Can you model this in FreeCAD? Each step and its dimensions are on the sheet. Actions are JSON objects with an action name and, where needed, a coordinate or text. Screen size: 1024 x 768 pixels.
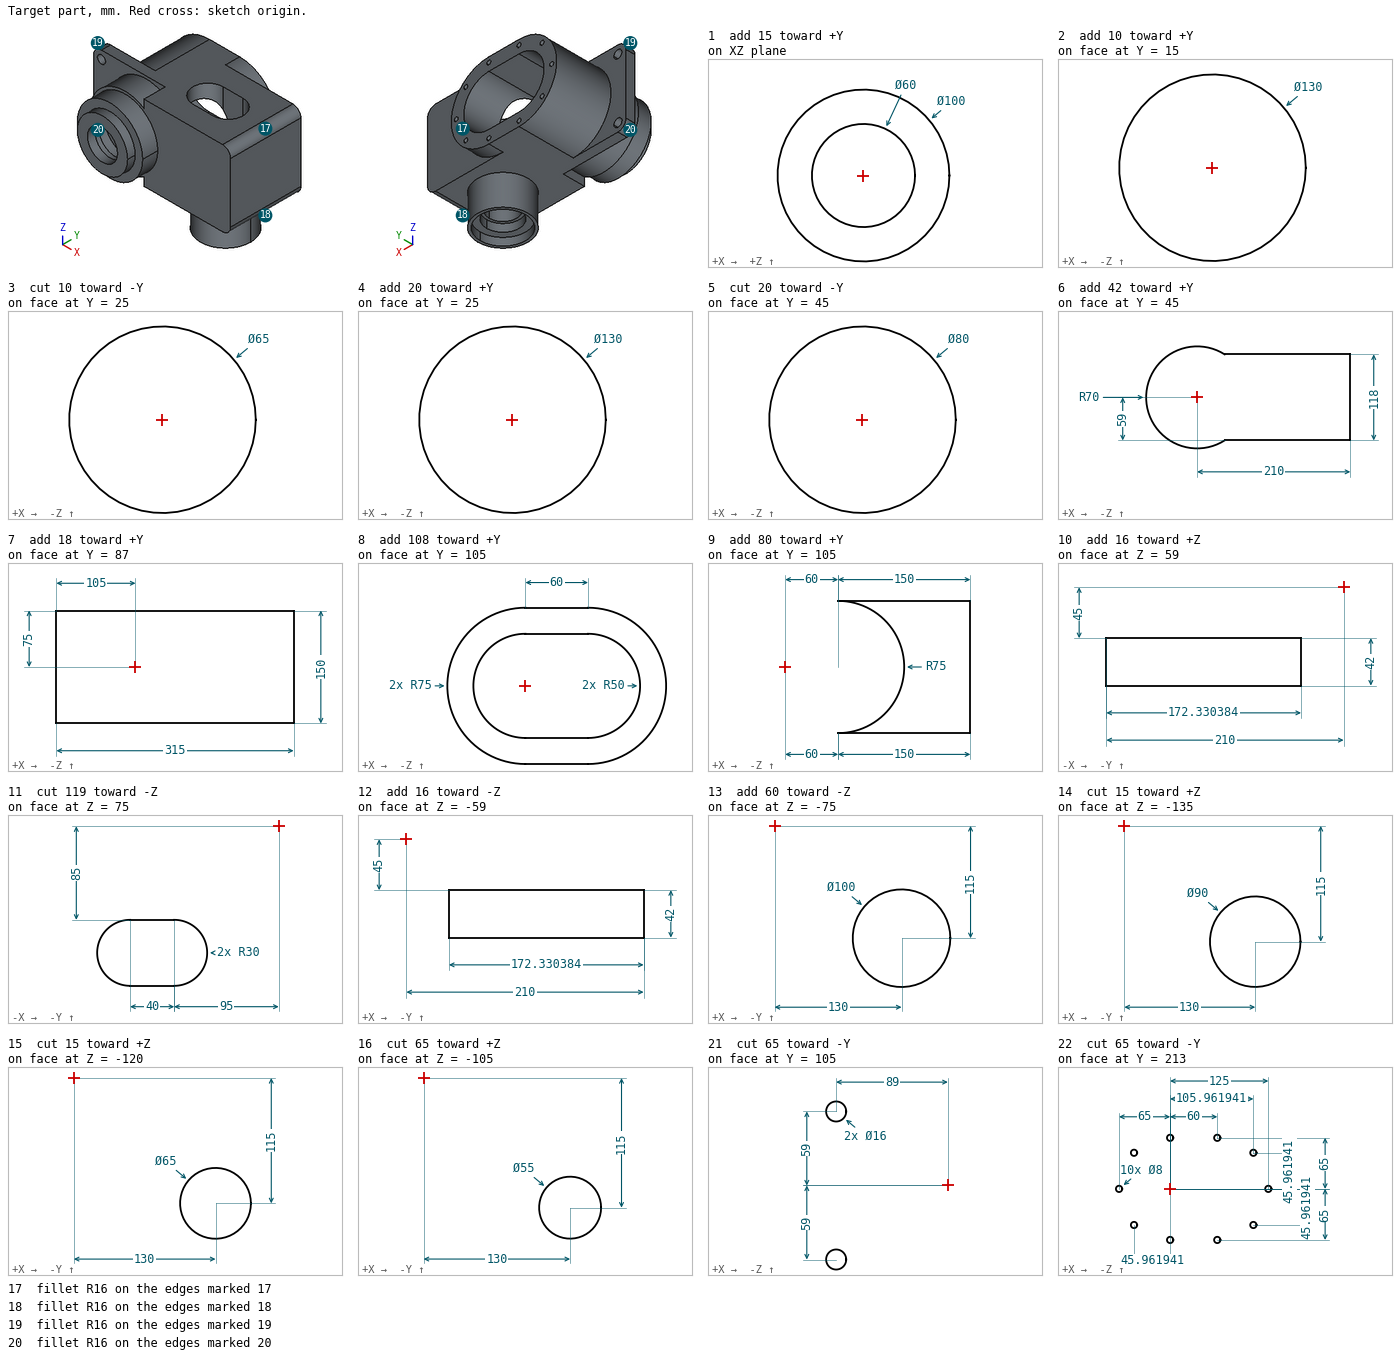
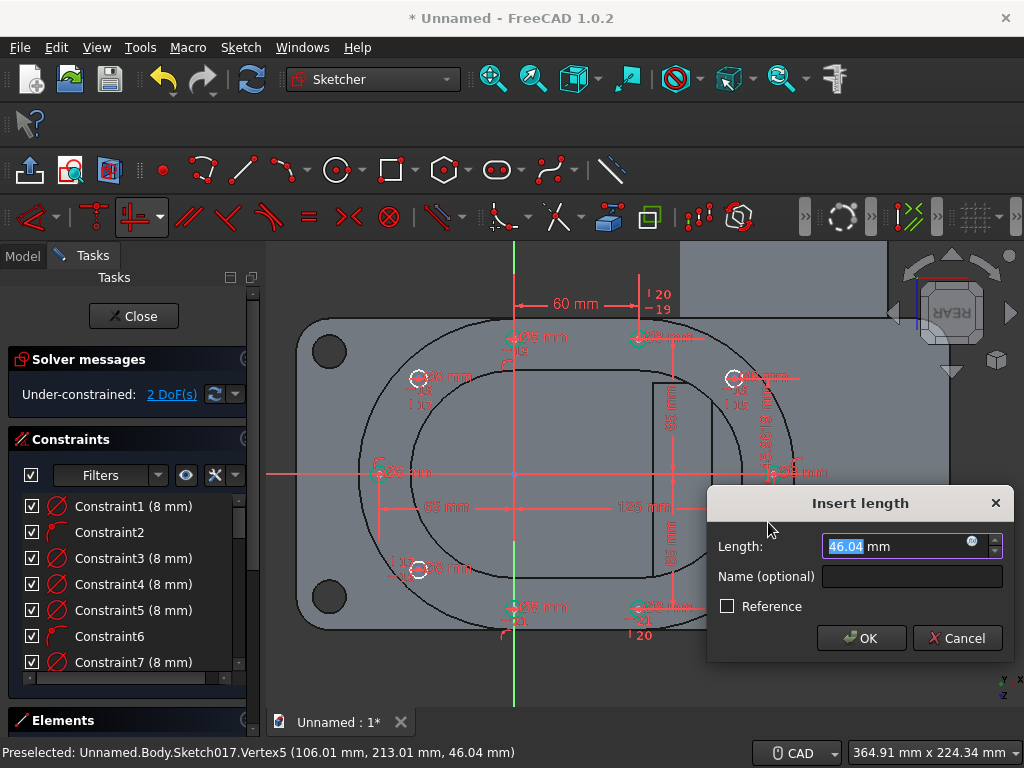
{"action": "type", "text": "45.961941"}
{"action": "key", "text": "Return"}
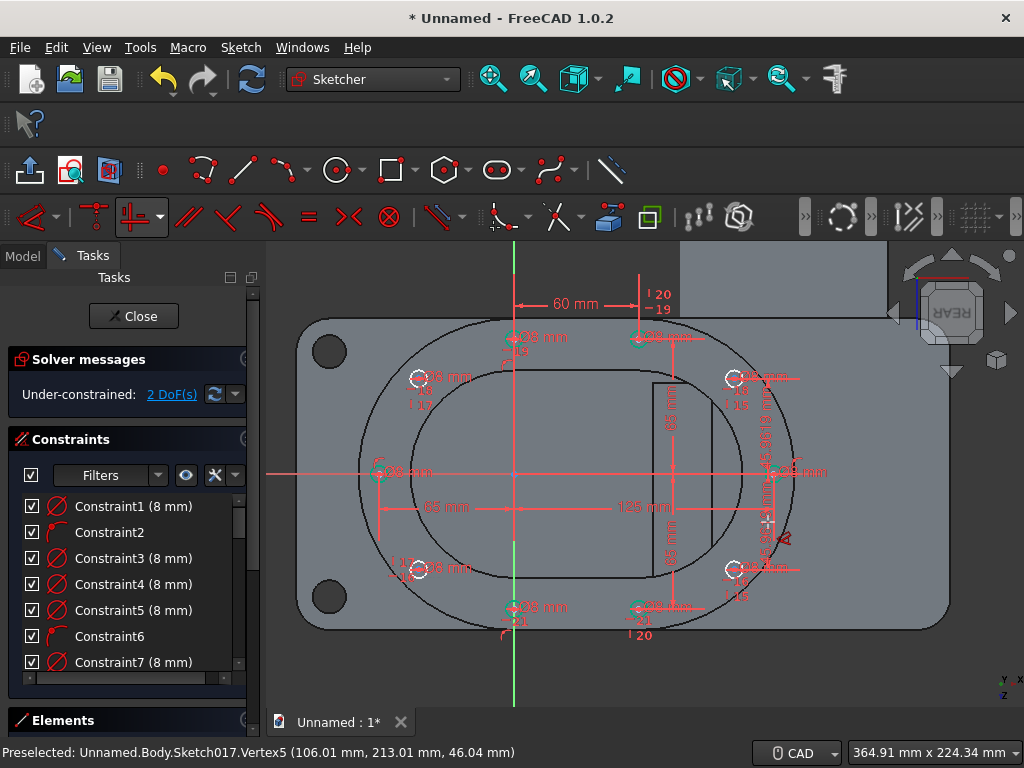
{"action": "left_click", "coordinate": [419, 570]}
{"action": "left_click", "coordinate": [466, 604]}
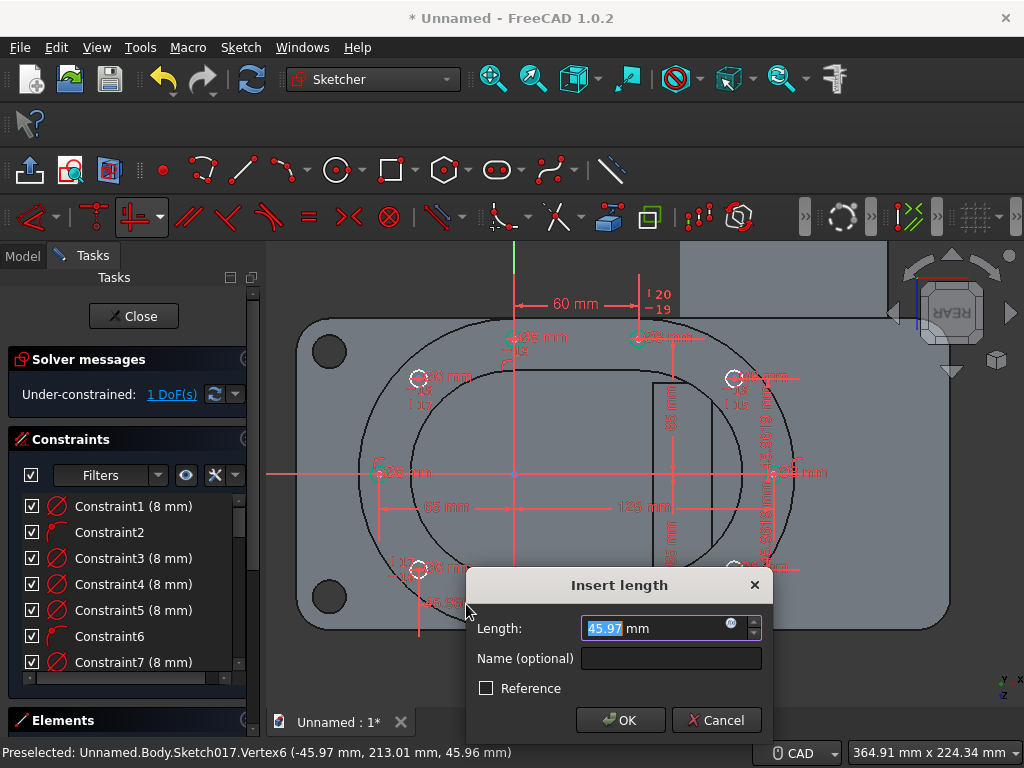
{"action": "type", "text": "45.961941"}
{"action": "key", "text": "Return"}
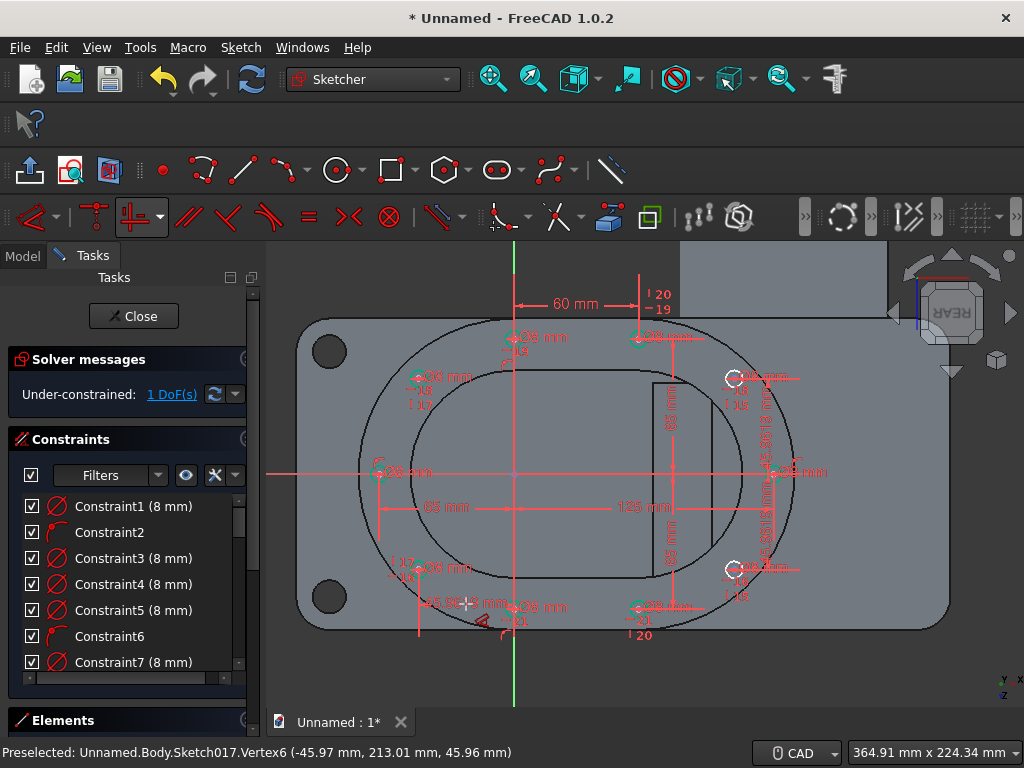
{"action": "left_click", "coordinate": [734, 379]}
{"action": "left_click", "coordinate": [574, 345]}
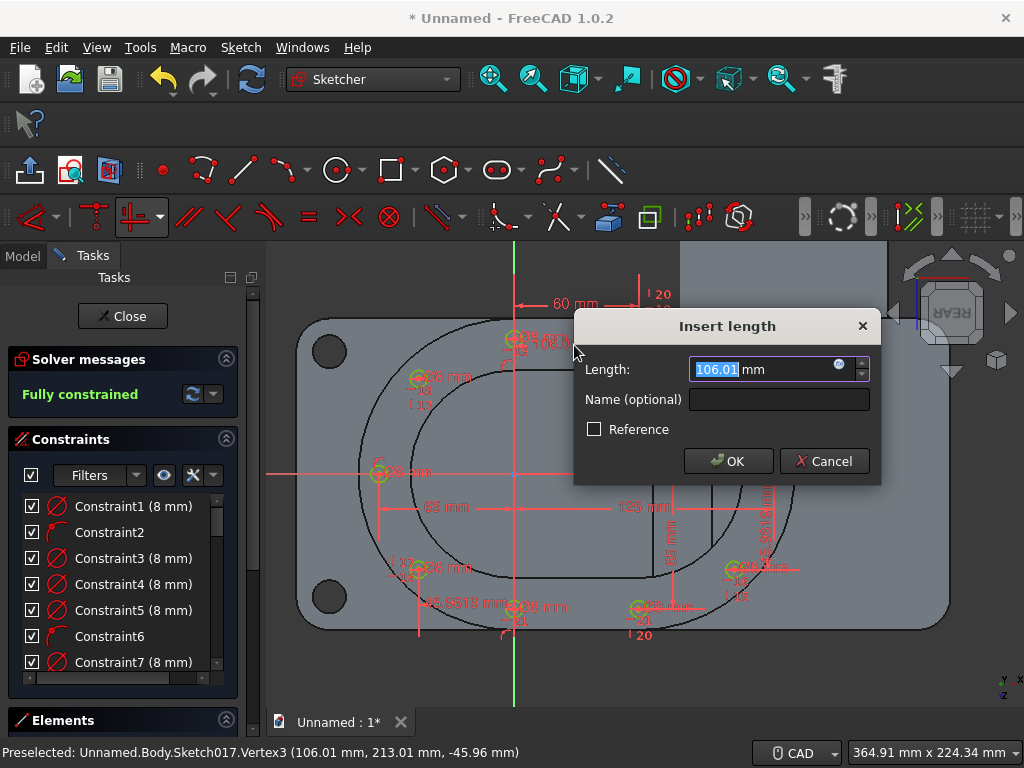
{"action": "type", "text": "105.961941"}
{"action": "key", "text": "Return"}
{"action": "key", "text": "Escape"}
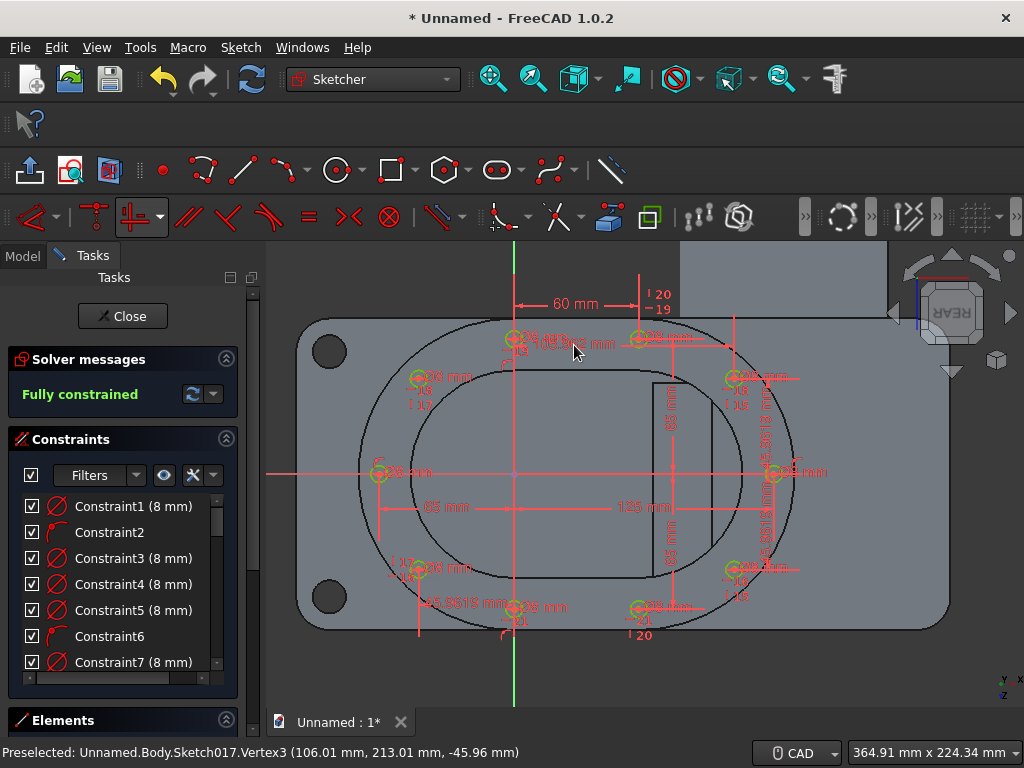
{"action": "left_click", "coordinate": [123, 316]}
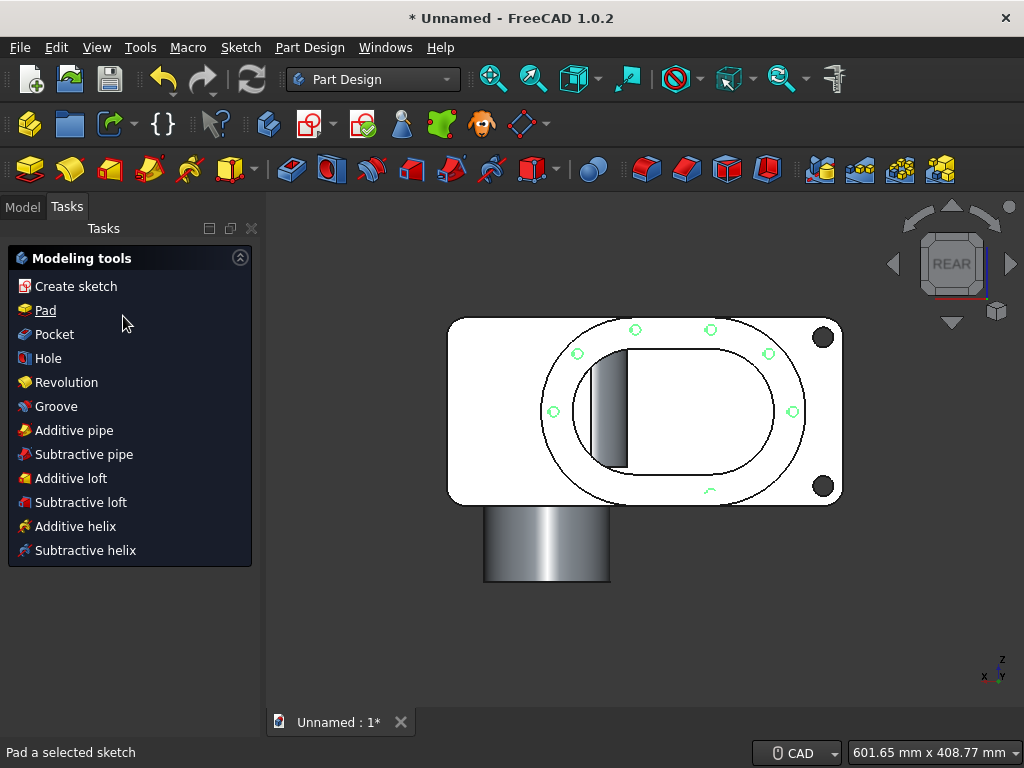
{"action": "left_click", "coordinate": [292, 170]}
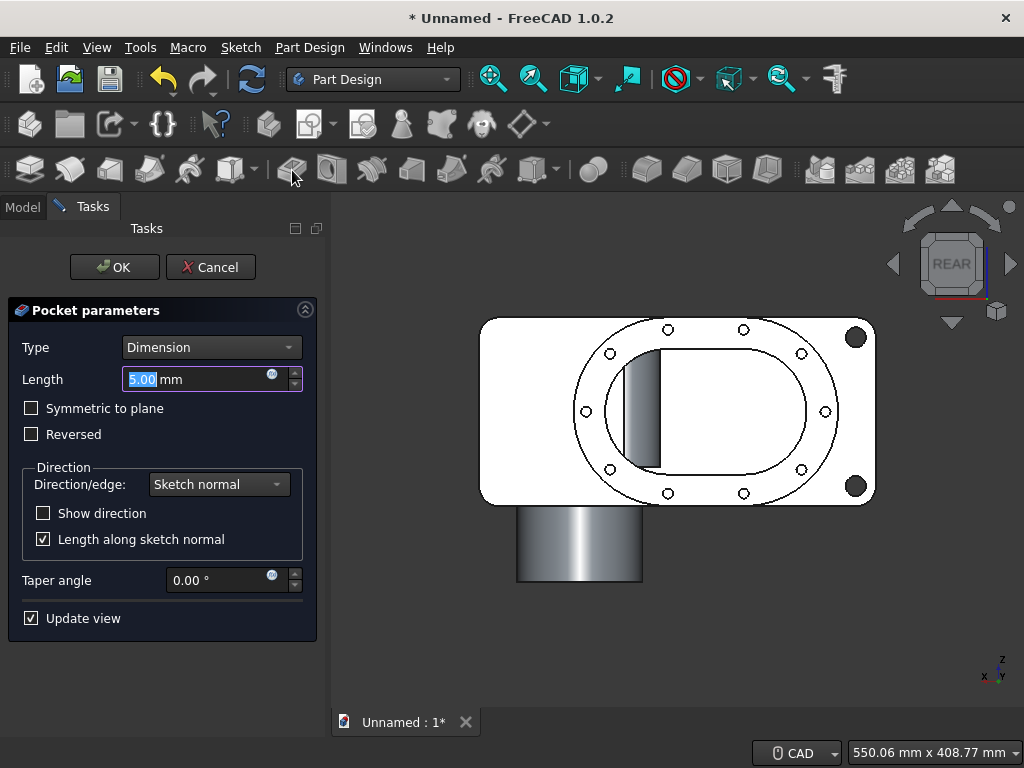
{"action": "type", "text": "65"}
{"action": "key", "text": "Tab"}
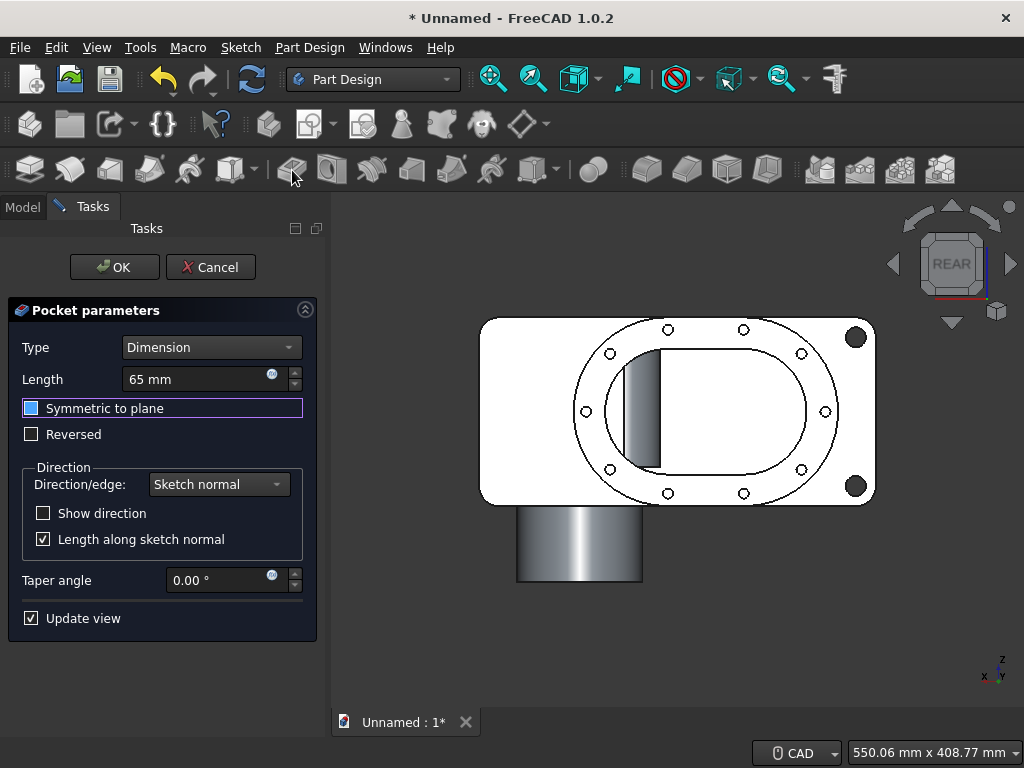
{"action": "left_click", "coordinate": [115, 267]}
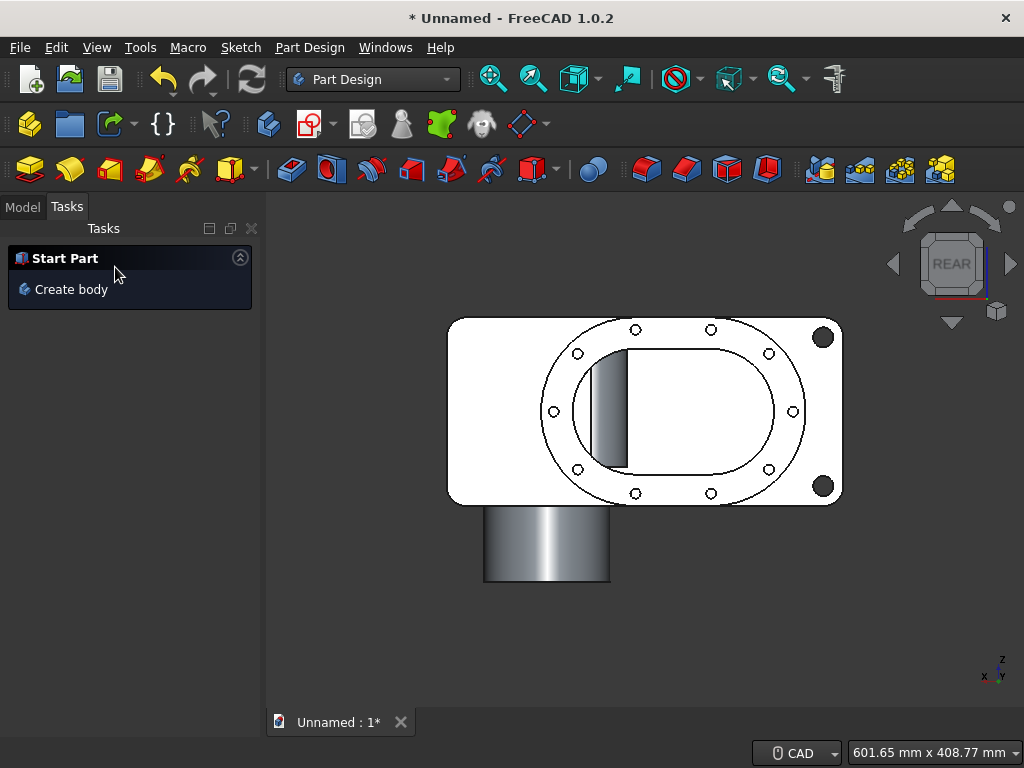
{"action": "key", "text": "0"}